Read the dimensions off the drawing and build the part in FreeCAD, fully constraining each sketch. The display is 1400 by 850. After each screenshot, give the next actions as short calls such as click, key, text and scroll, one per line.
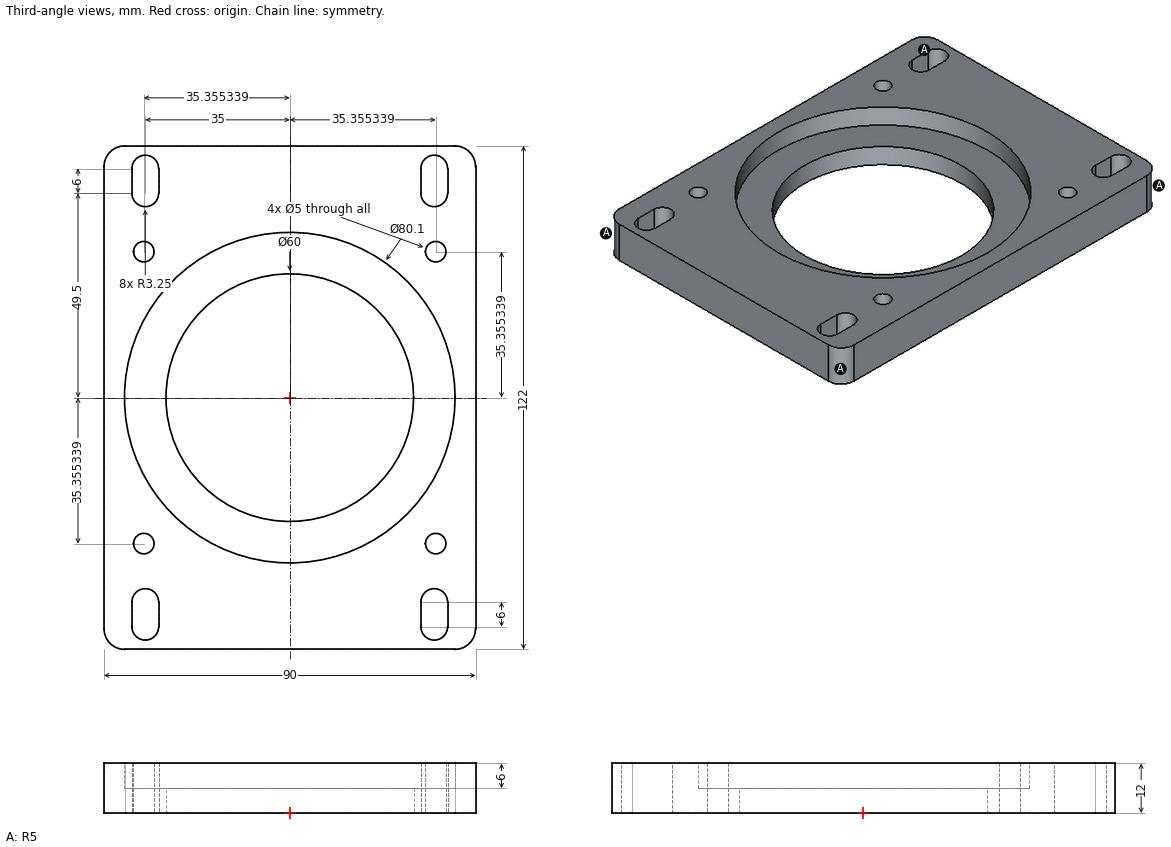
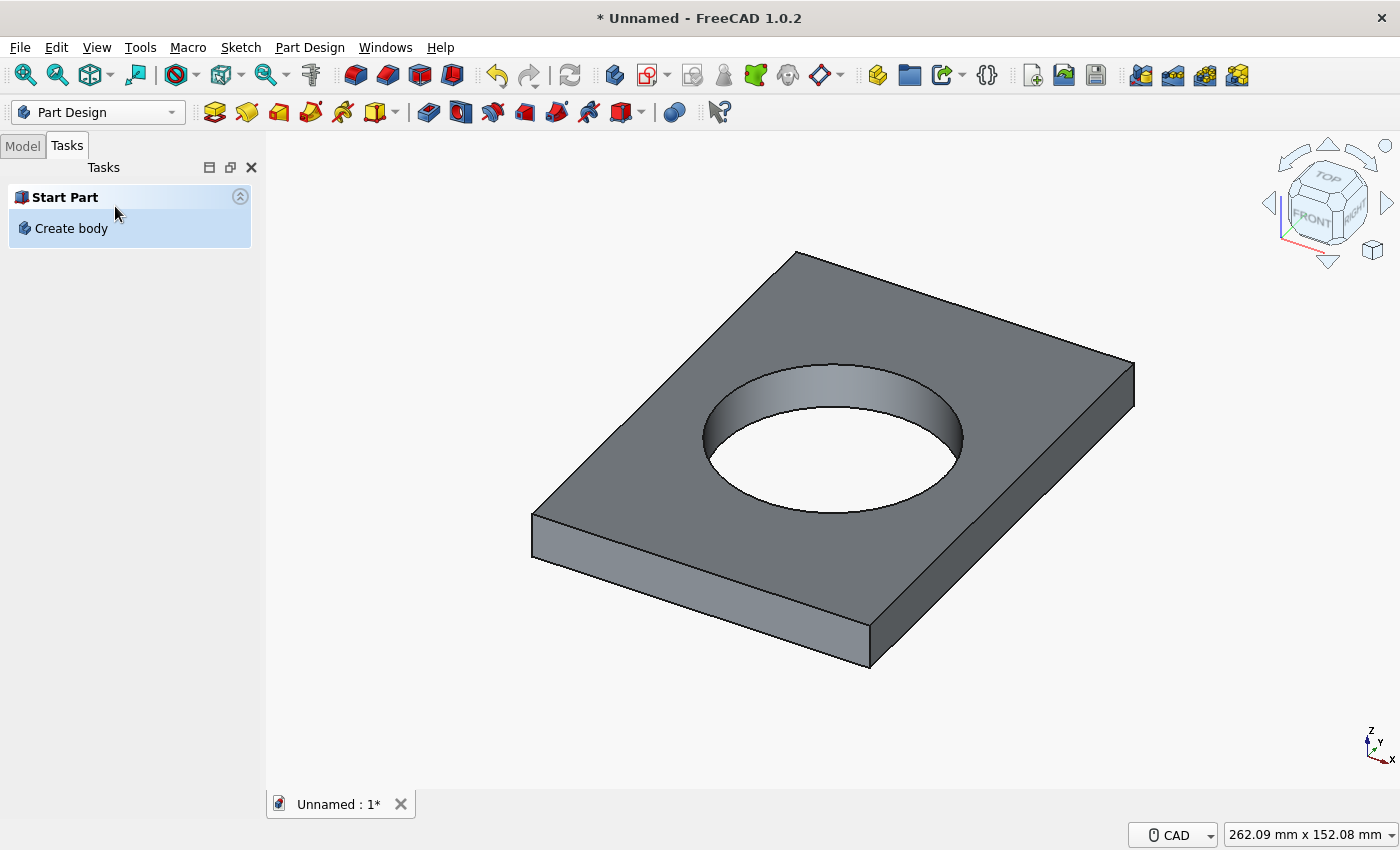
click(812, 331)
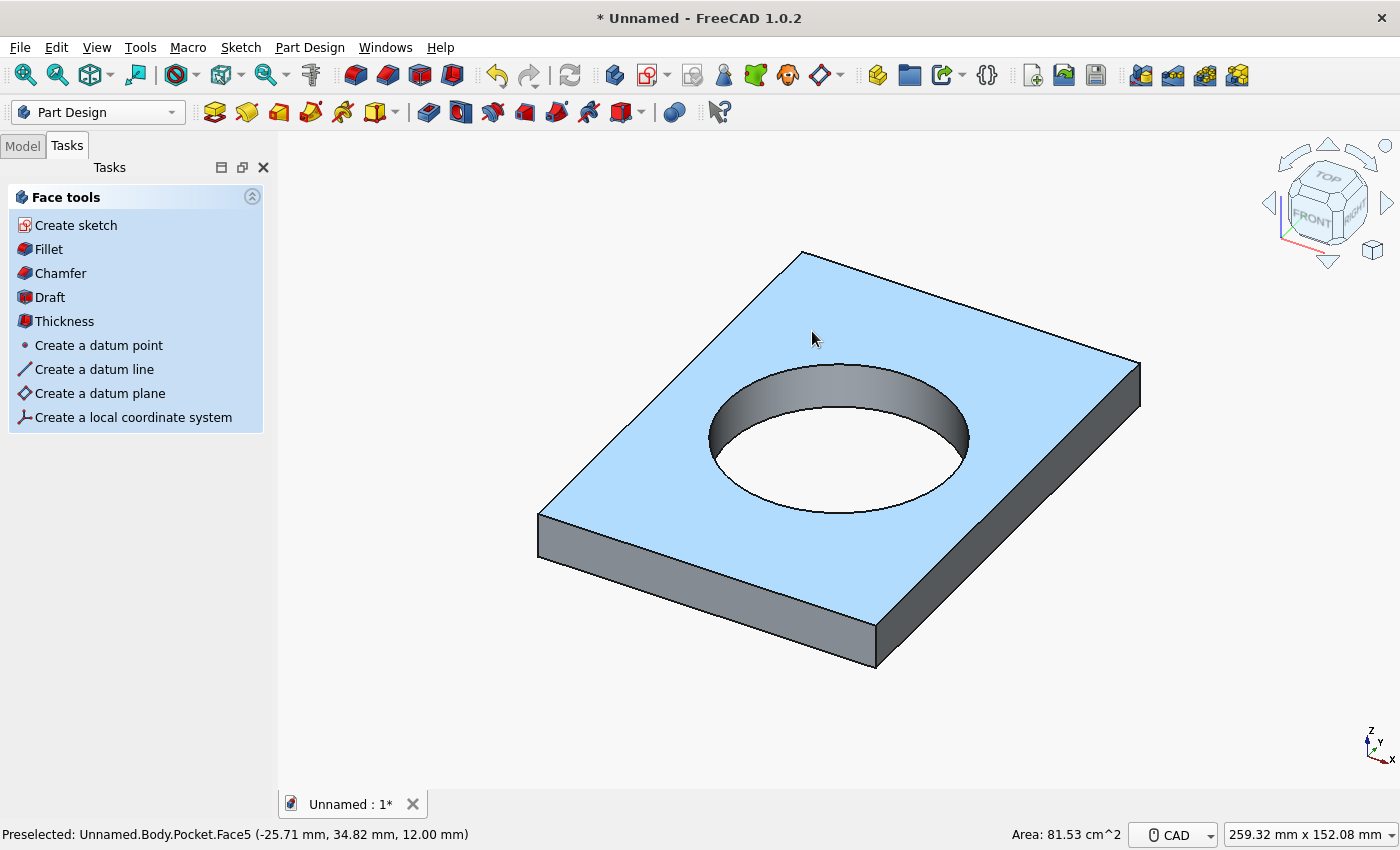
click(648, 76)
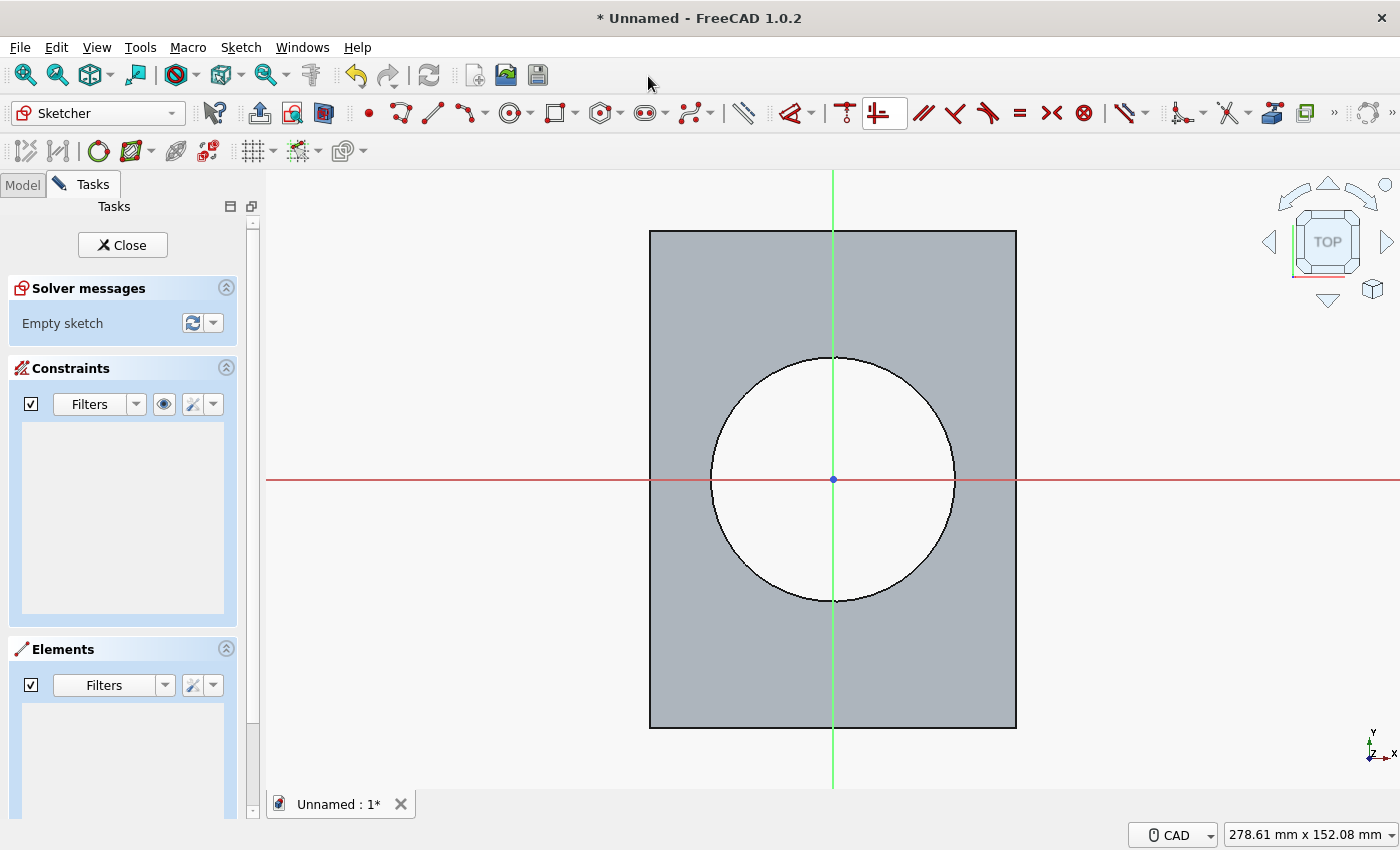
click(510, 114)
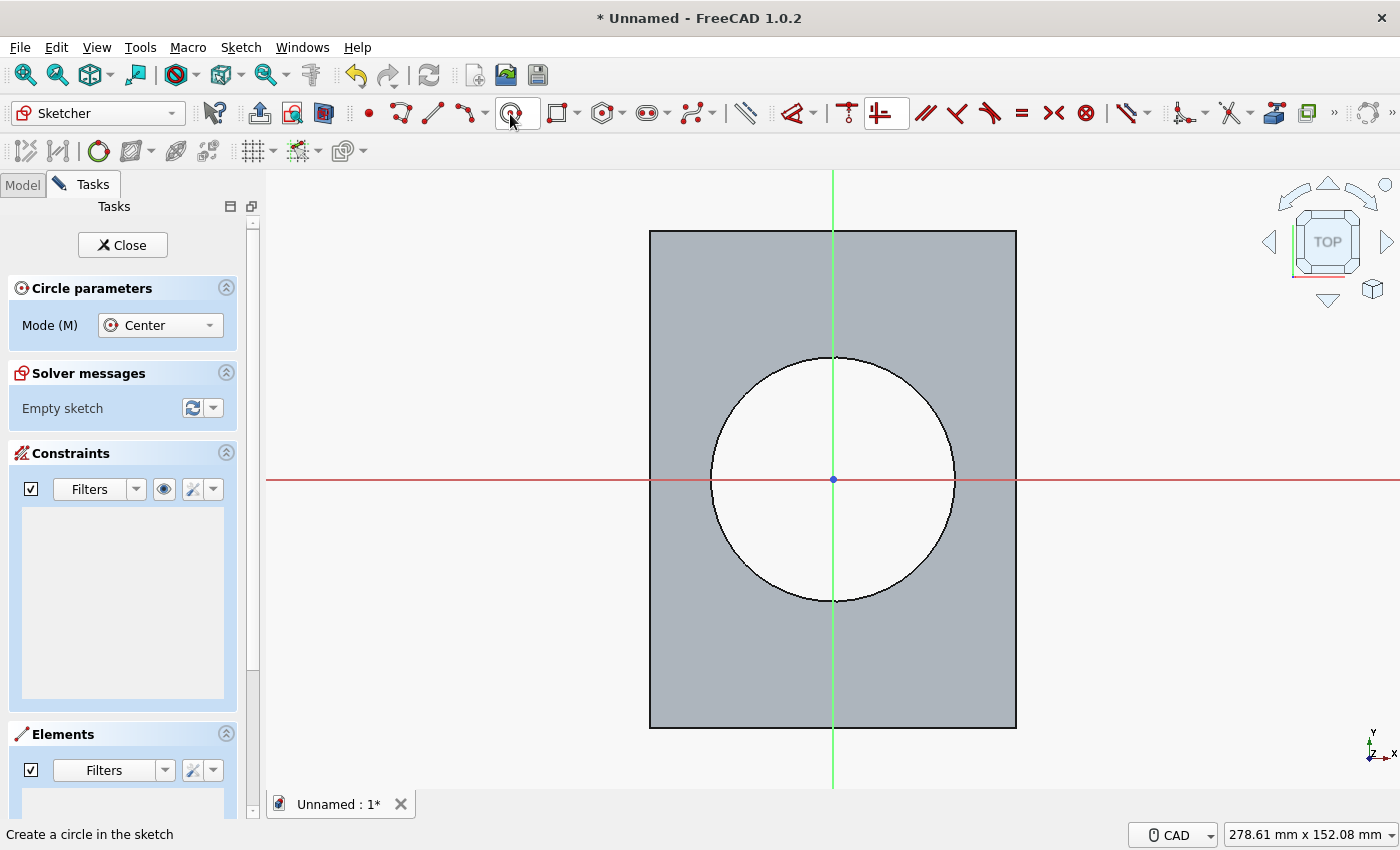
click(833, 480)
move(948, 364)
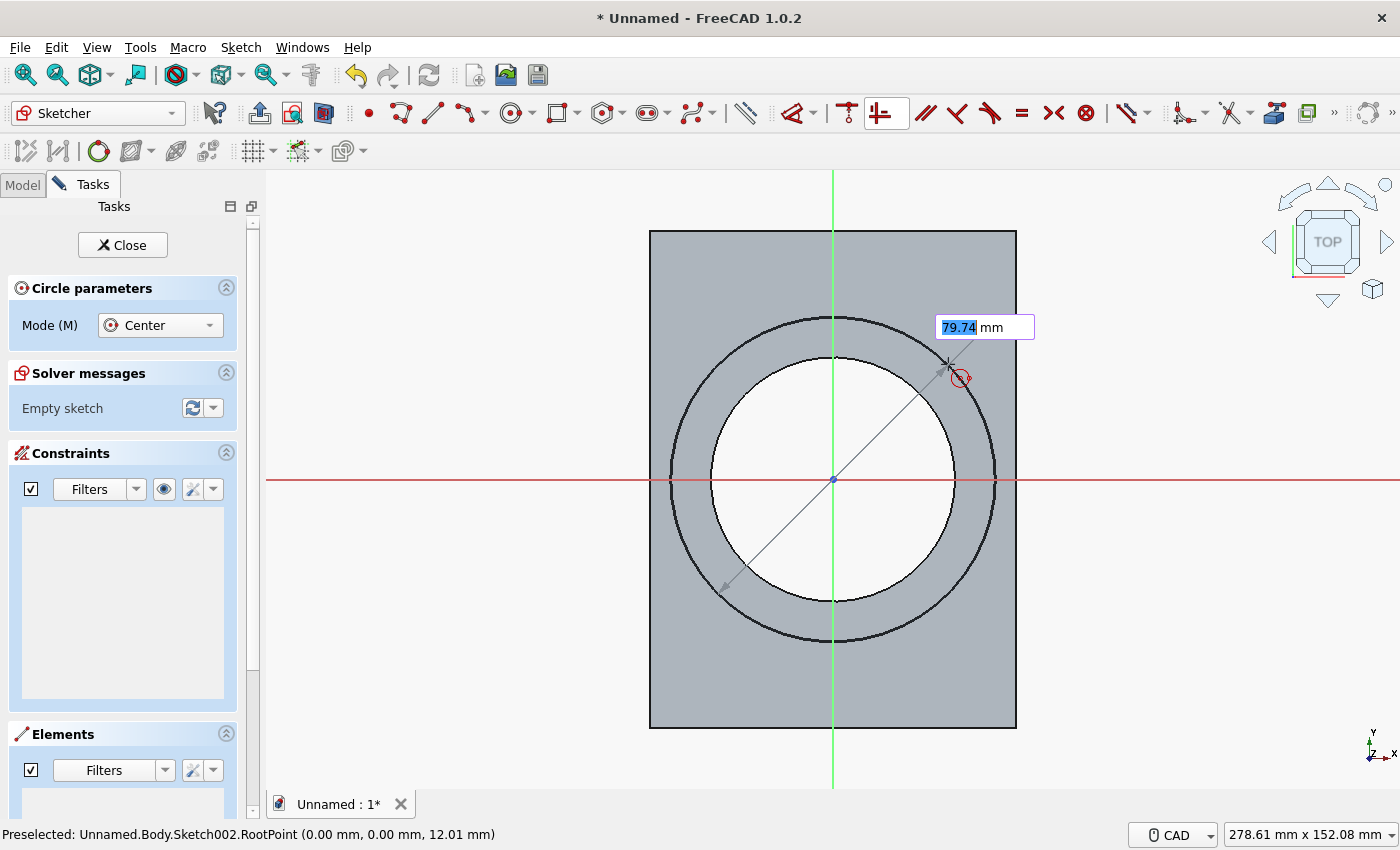
text(80.1)
key(Return)
key(Escape)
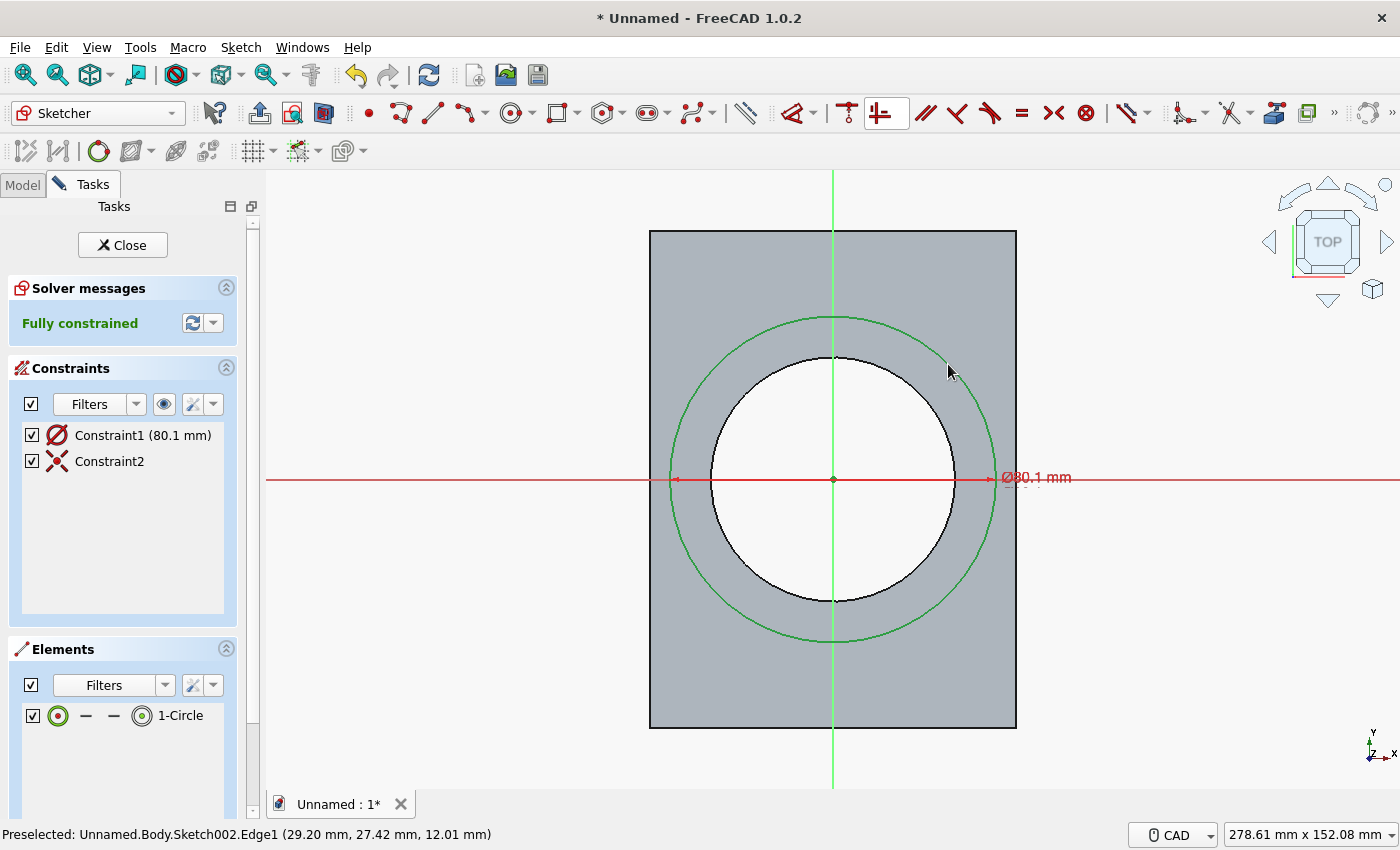
click(123, 245)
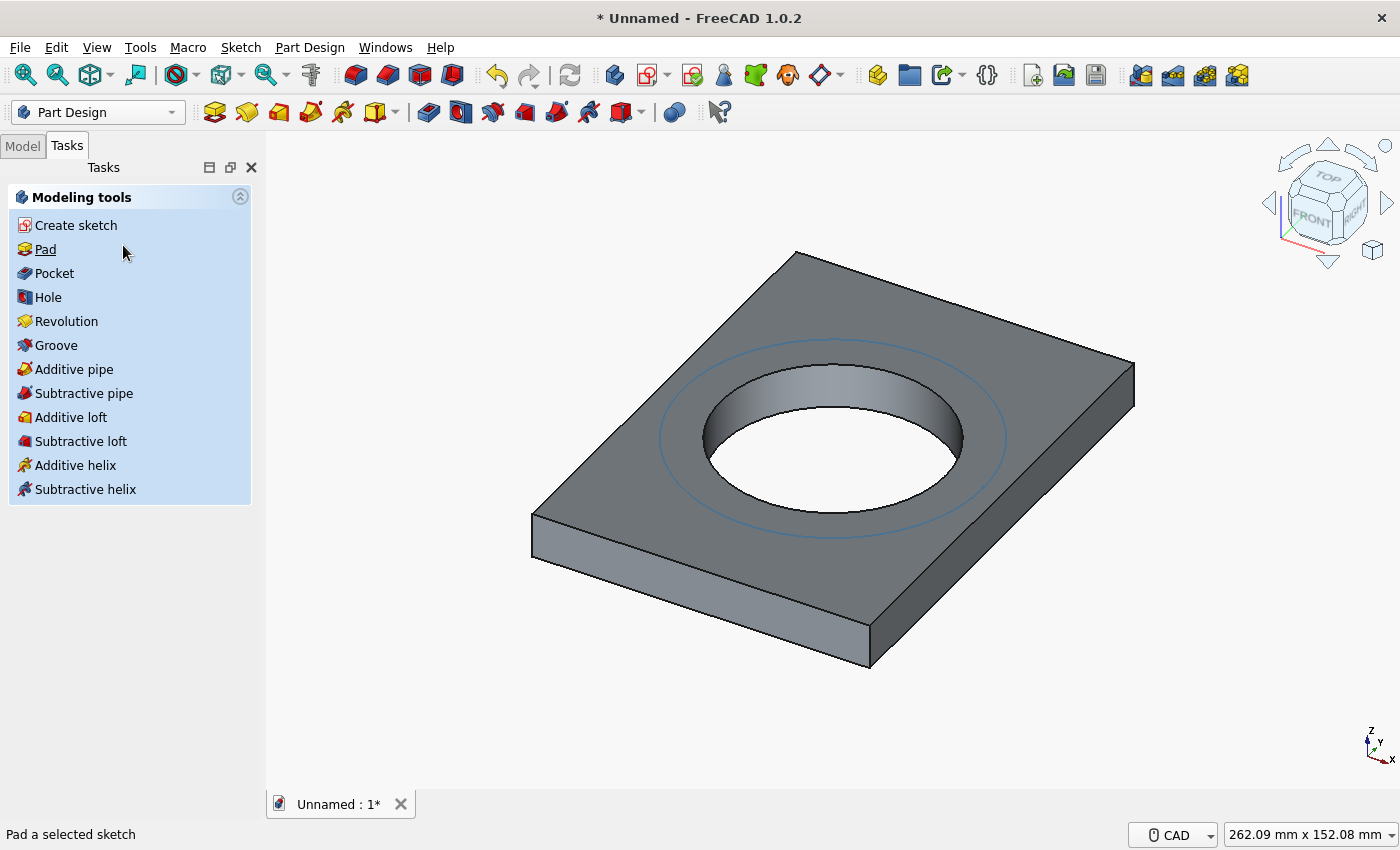
click(430, 112)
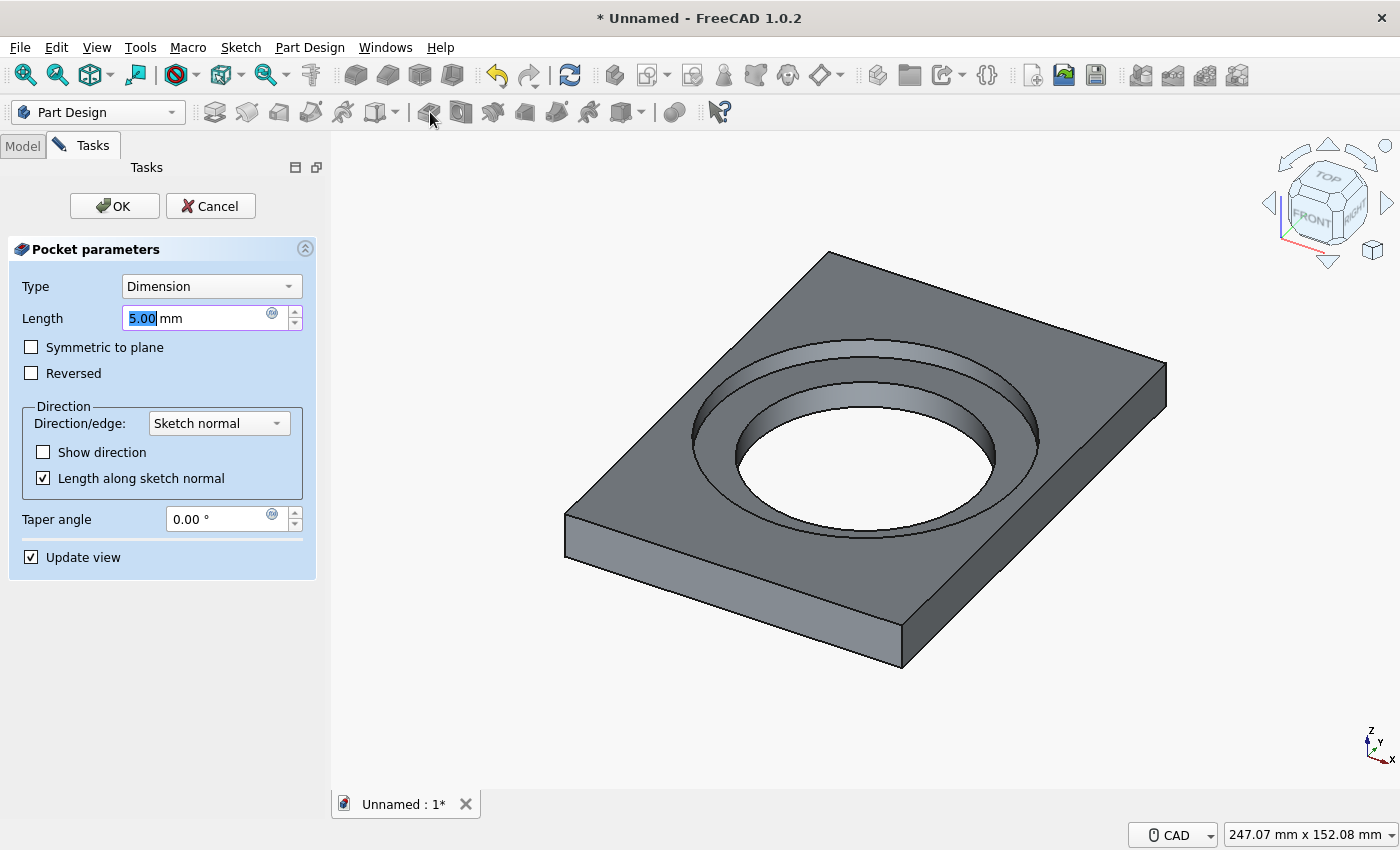
text(6)
key(Tab)